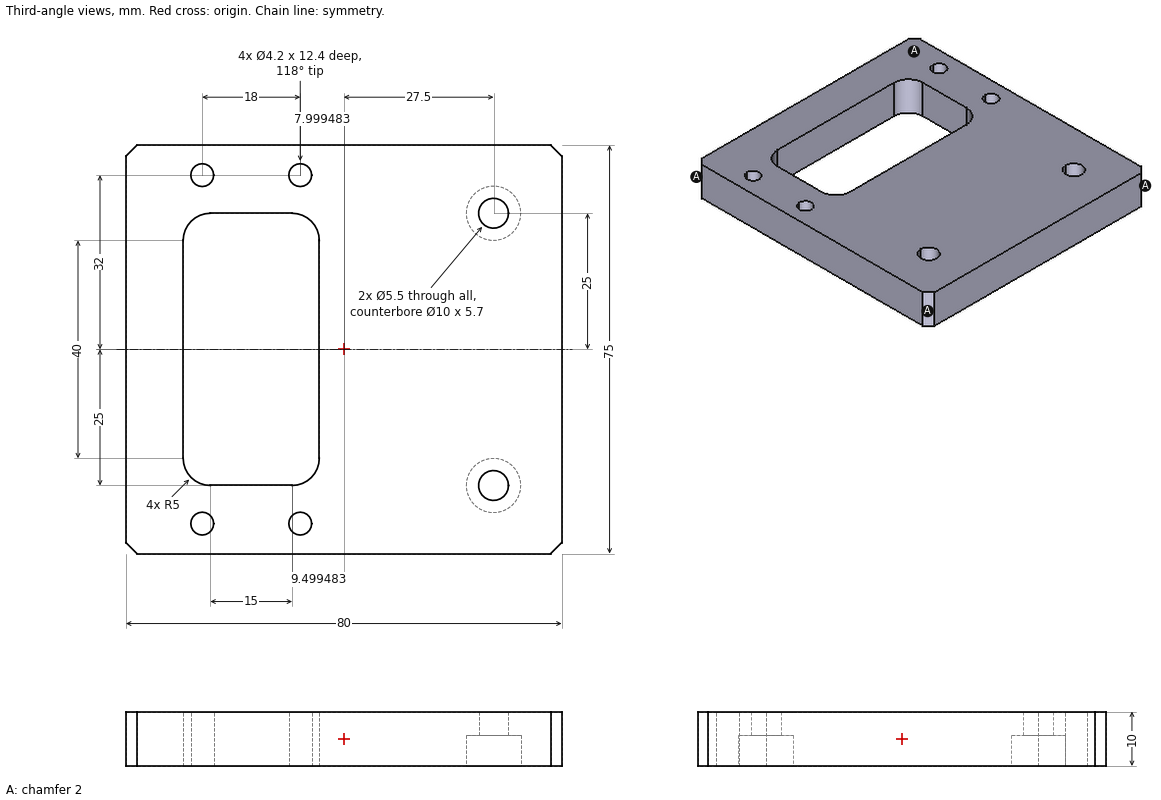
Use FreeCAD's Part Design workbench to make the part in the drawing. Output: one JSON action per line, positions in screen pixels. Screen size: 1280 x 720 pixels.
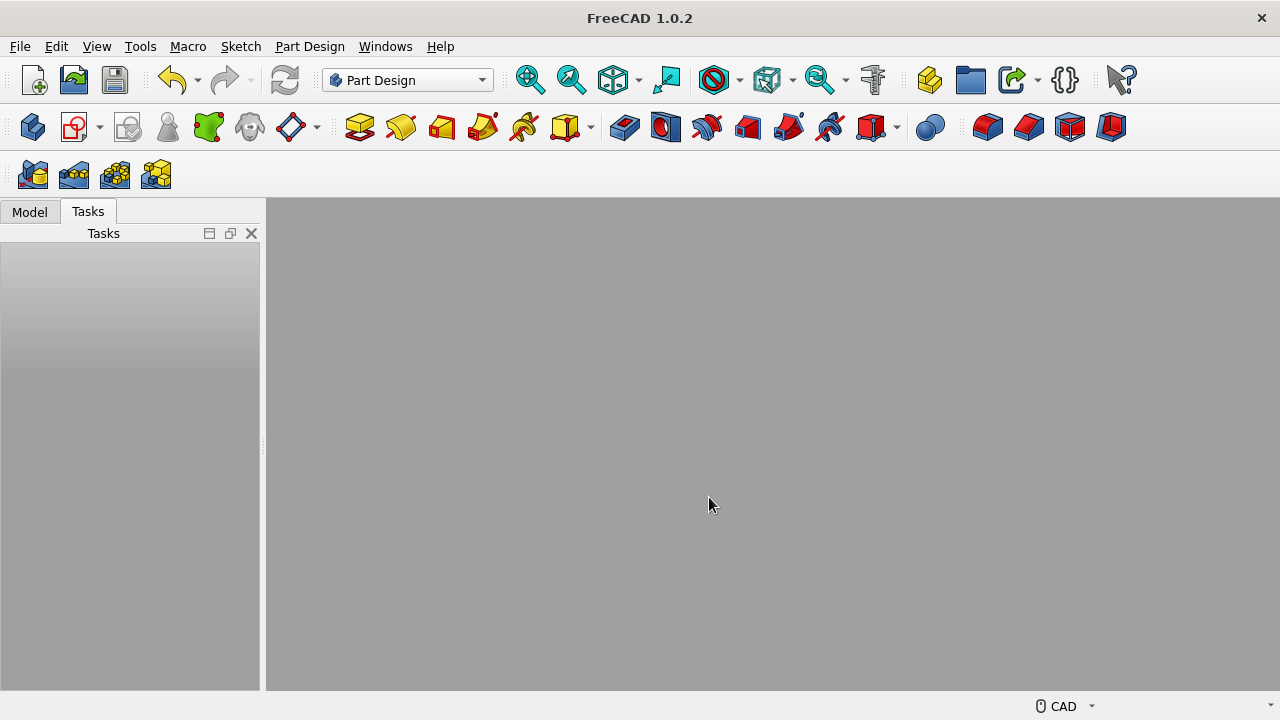
{"action": "key", "text": "ctrl+n"}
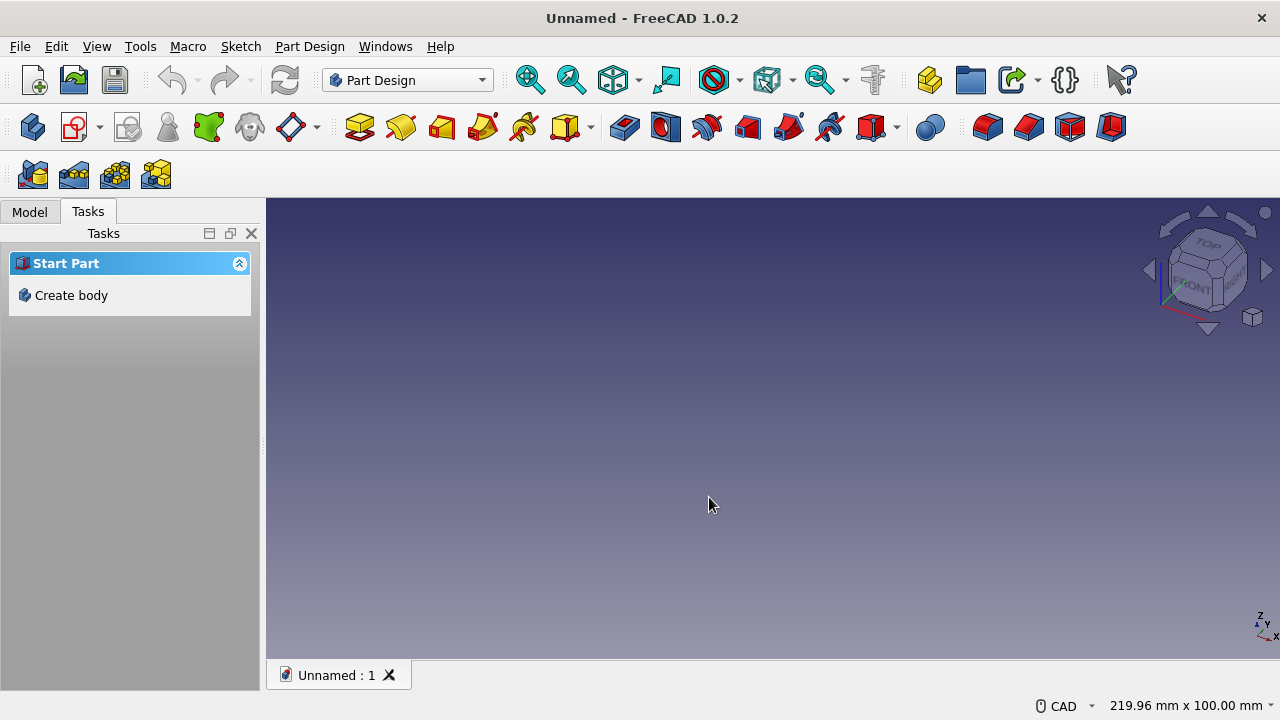
{"action": "left_click", "coordinate": [74, 128]}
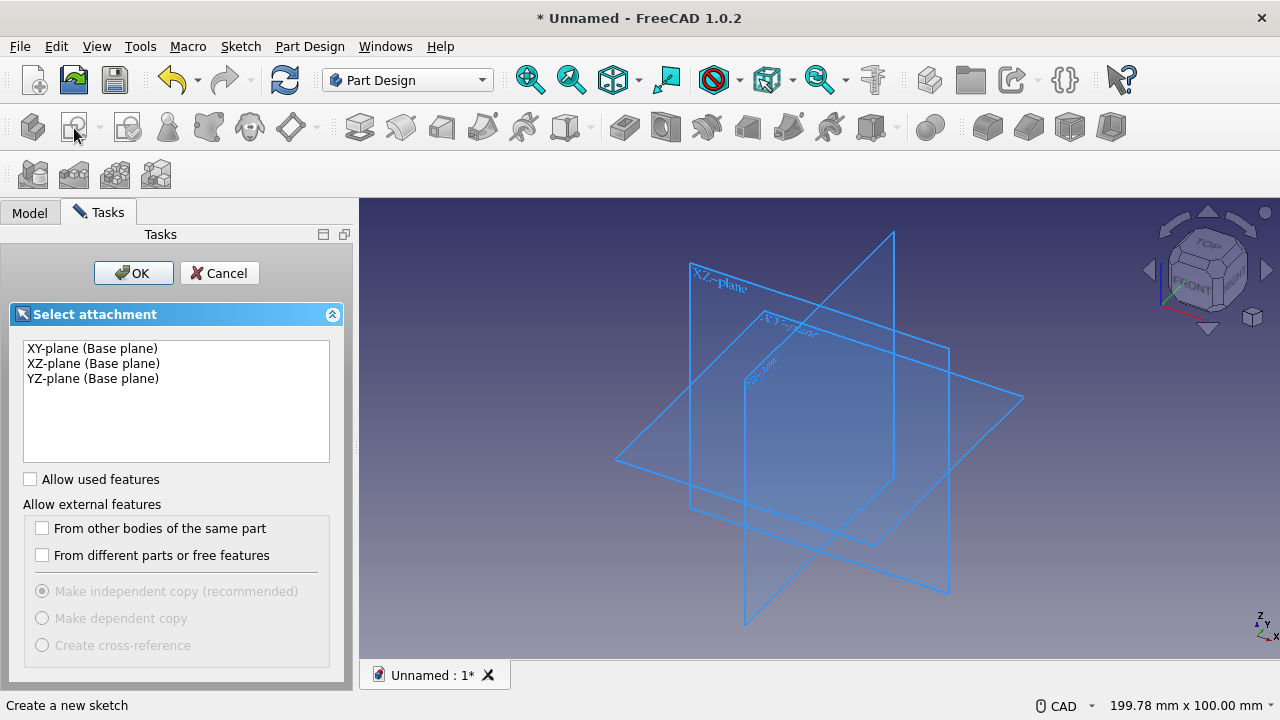
{"action": "left_click", "coordinate": [84, 348]}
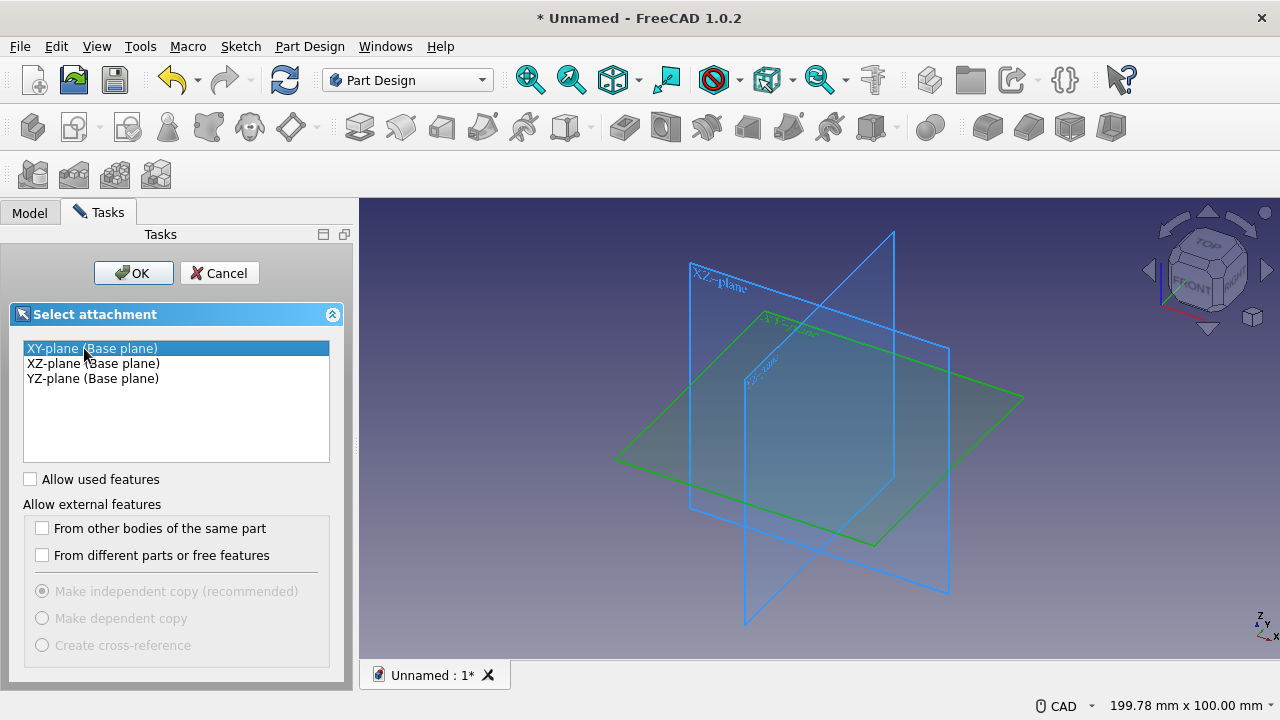
{"action": "left_click", "coordinate": [134, 273]}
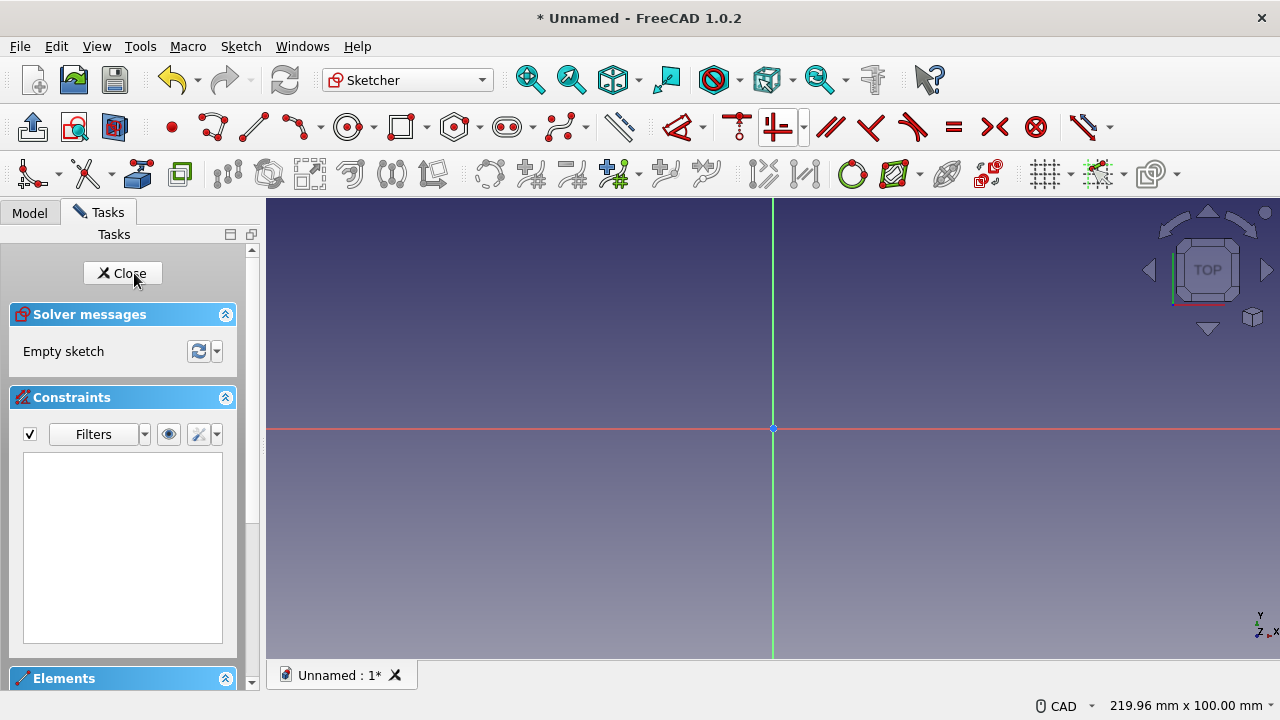
{"action": "key", "text": "g v"}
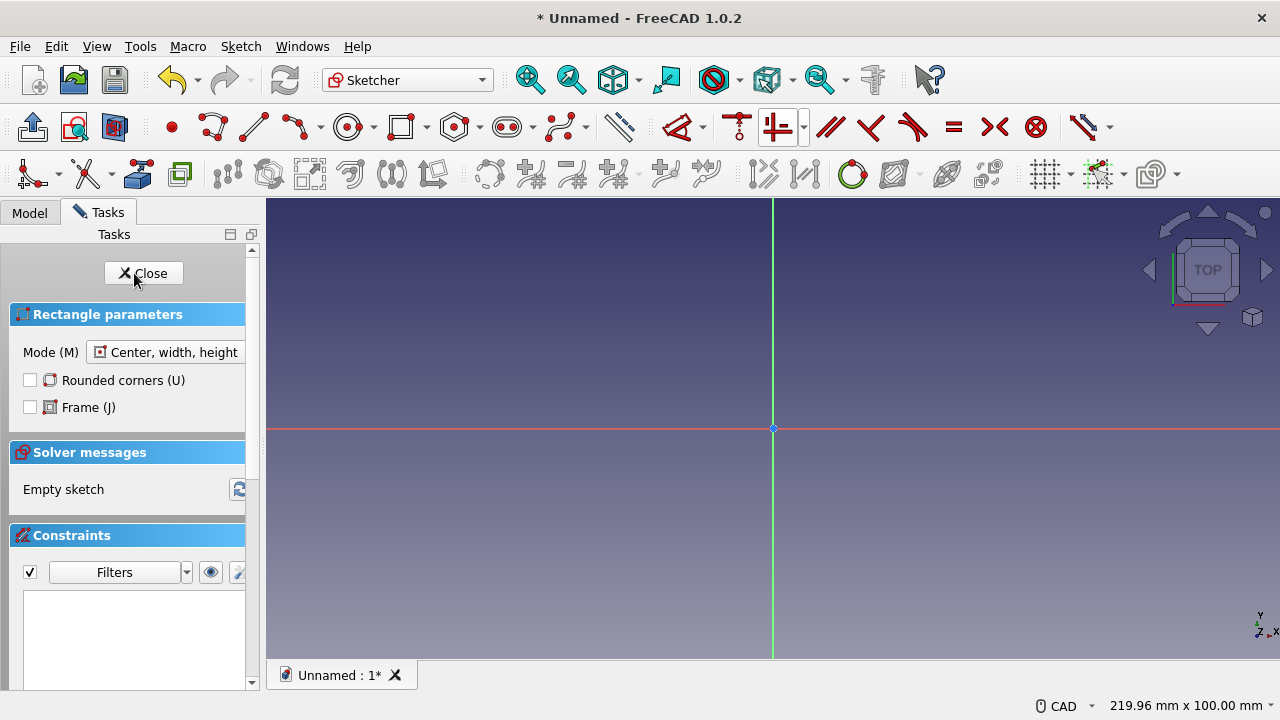
{"action": "left_click", "coordinate": [773, 428]}
{"action": "mouse_move", "coordinate": [957, 256]}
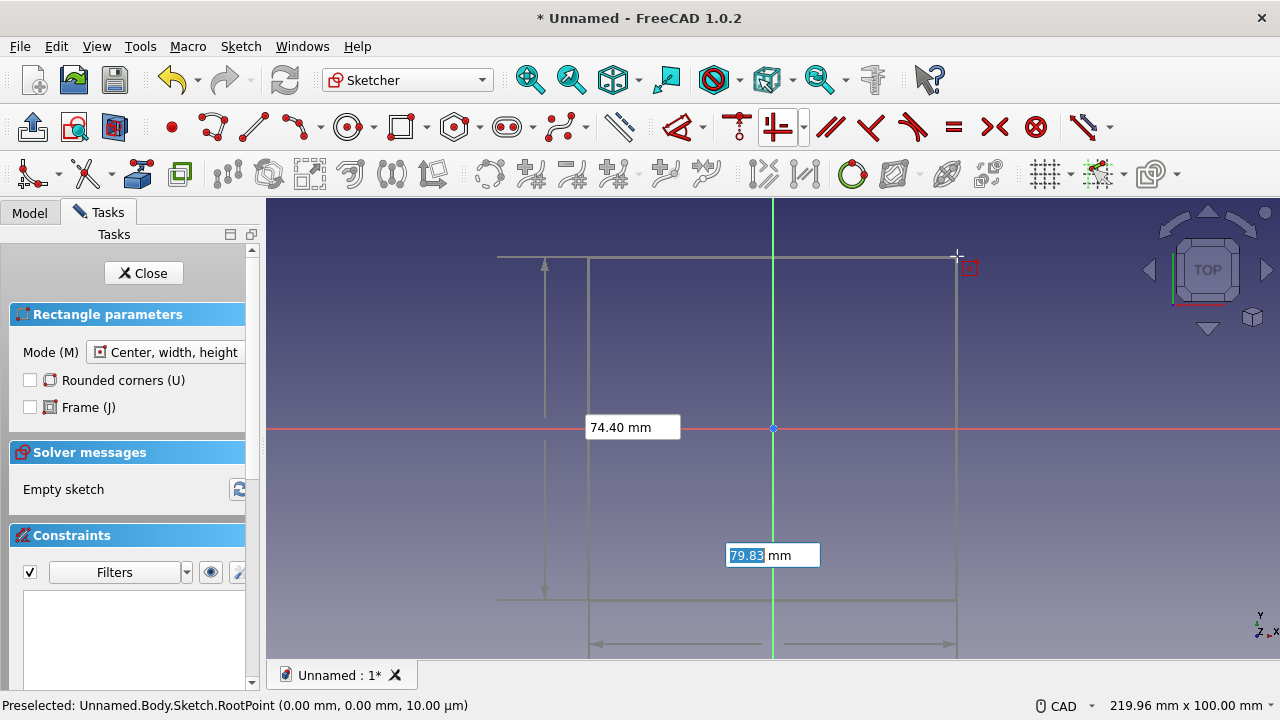
{"action": "type", "text": "80"}
{"action": "key", "text": "Tab"}
{"action": "type", "text": "75"}
{"action": "key", "text": "Return"}
{"action": "key", "text": "Escape"}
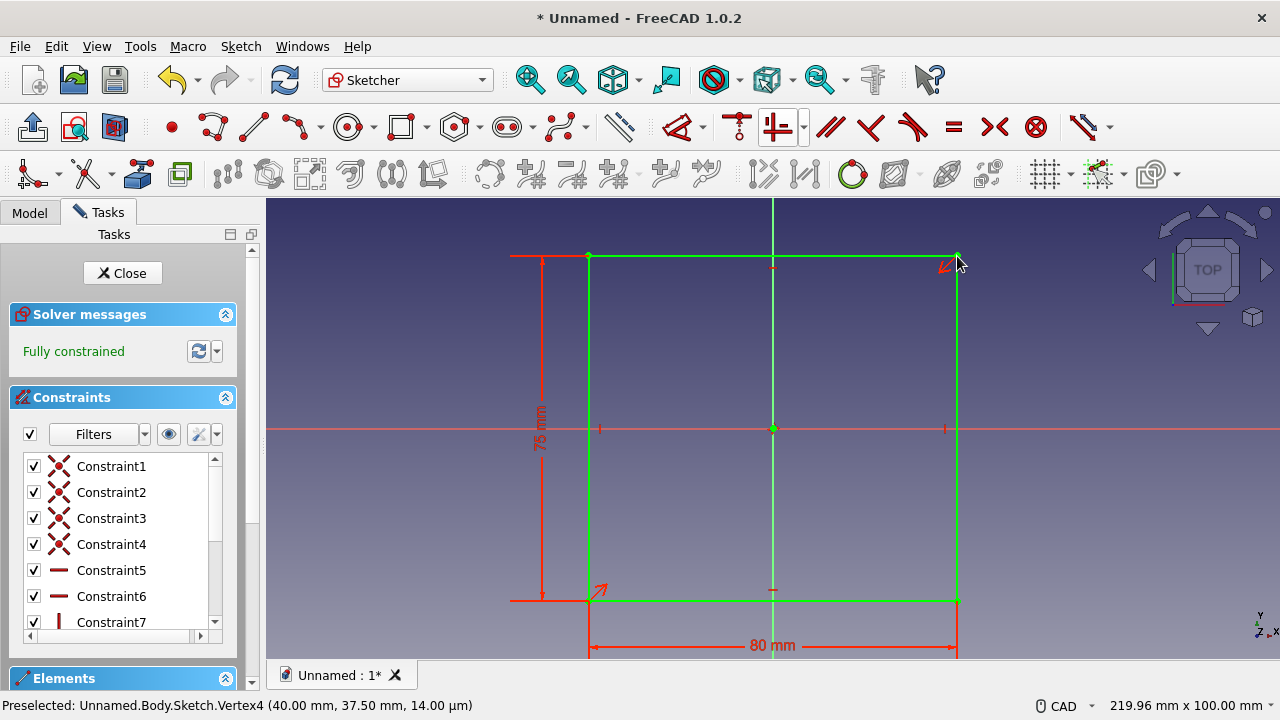
{"action": "left_click", "coordinate": [123, 273]}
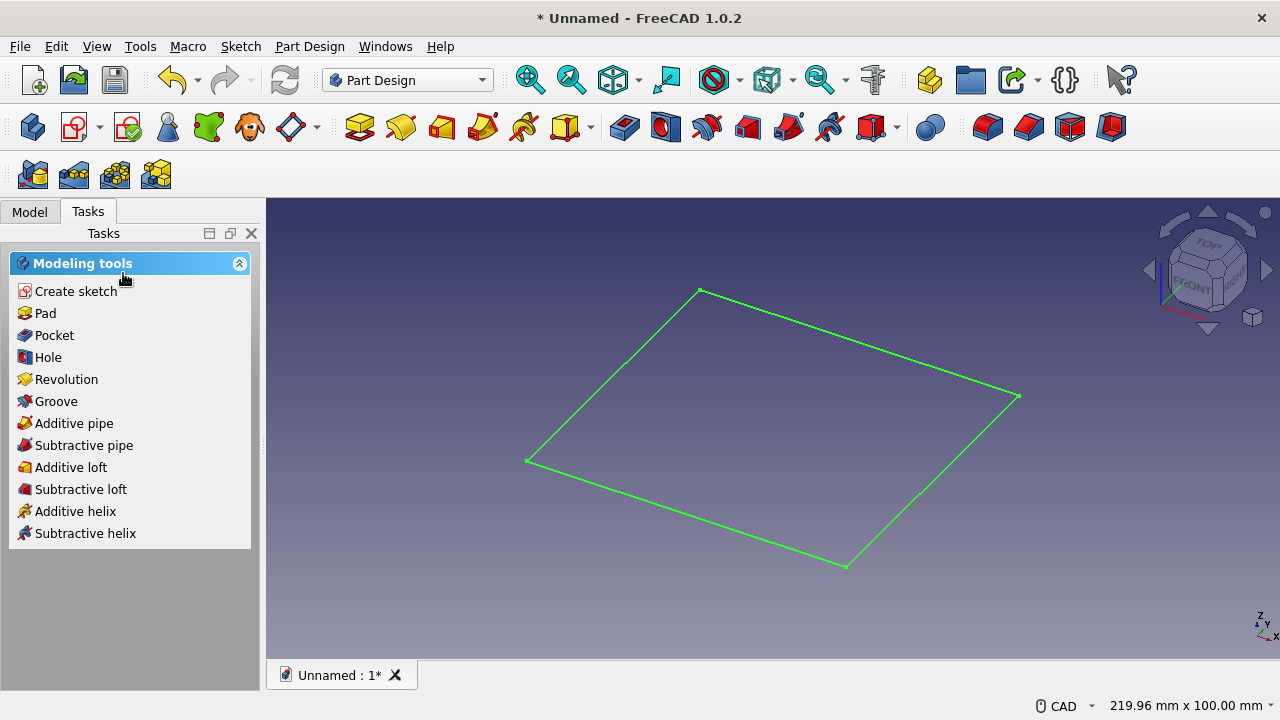
{"action": "left_click", "coordinate": [360, 128]}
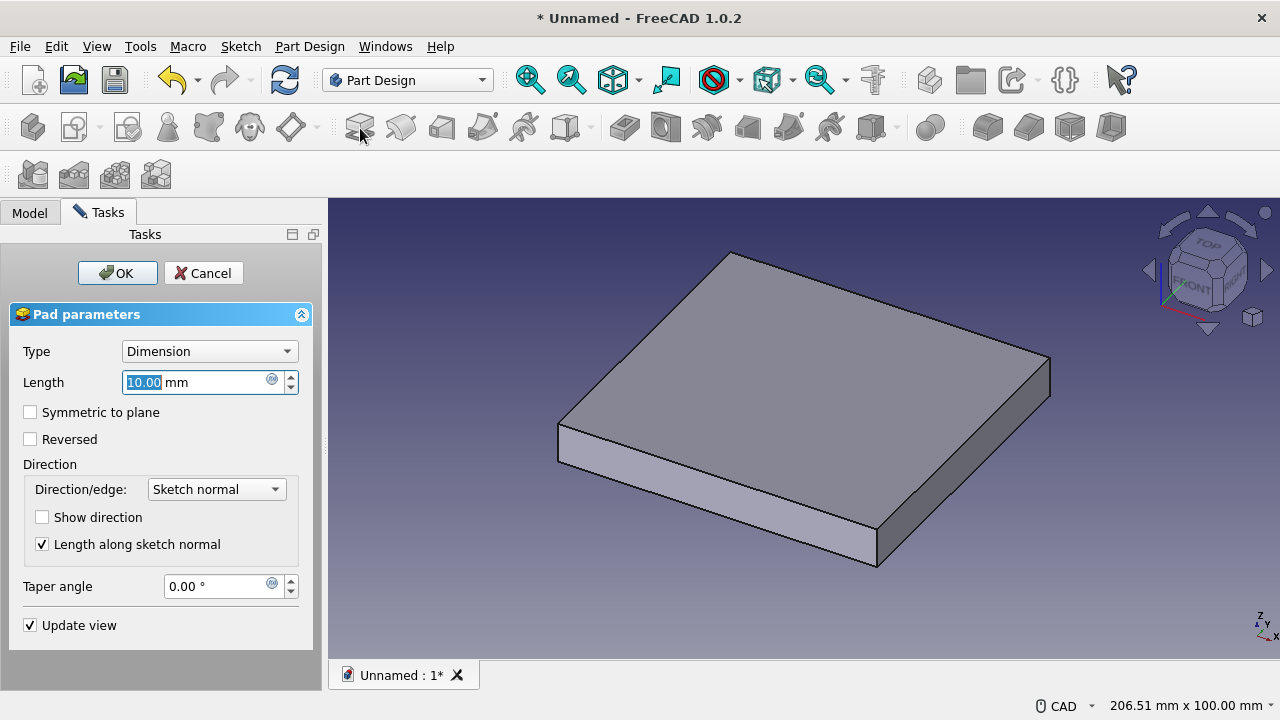
{"action": "type", "text": "10"}
{"action": "key", "text": "Tab"}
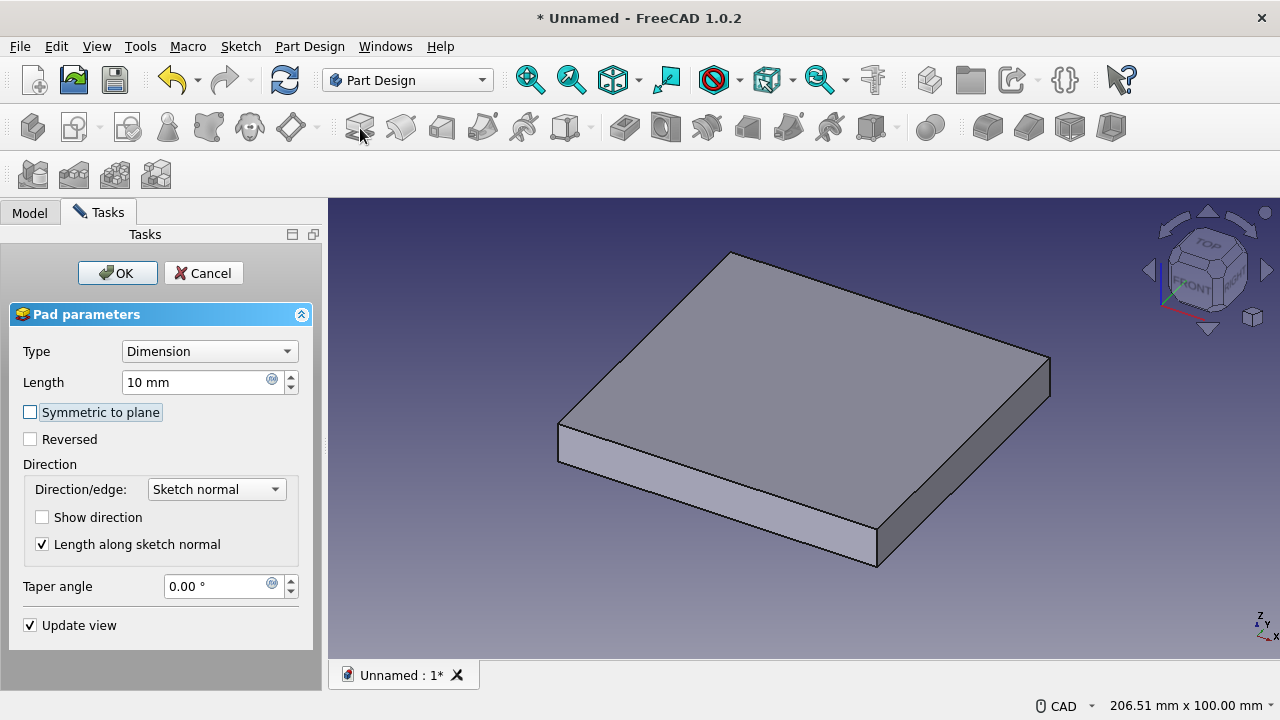
{"action": "left_click", "coordinate": [31, 412]}